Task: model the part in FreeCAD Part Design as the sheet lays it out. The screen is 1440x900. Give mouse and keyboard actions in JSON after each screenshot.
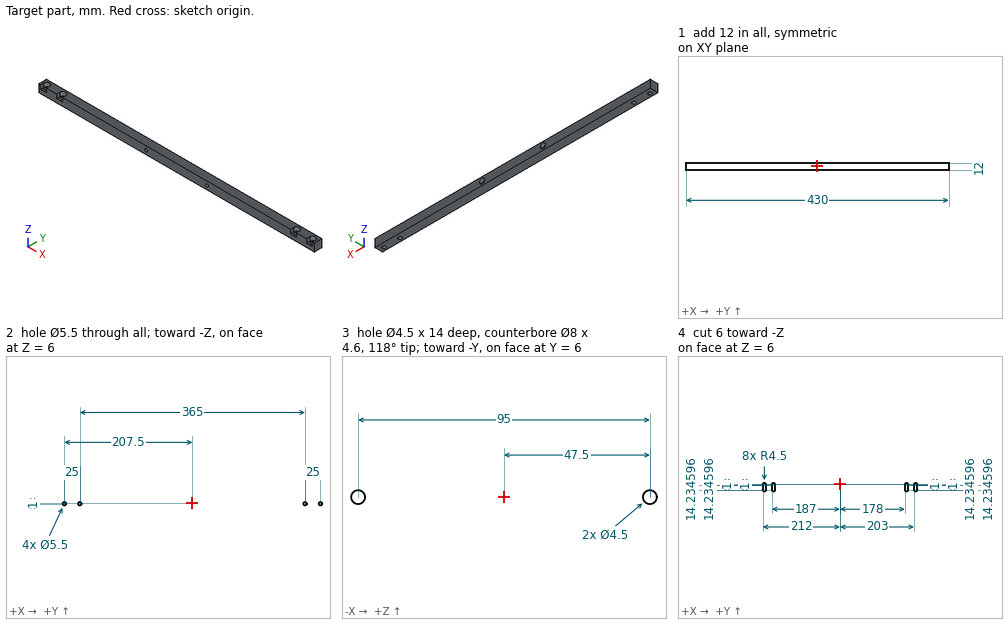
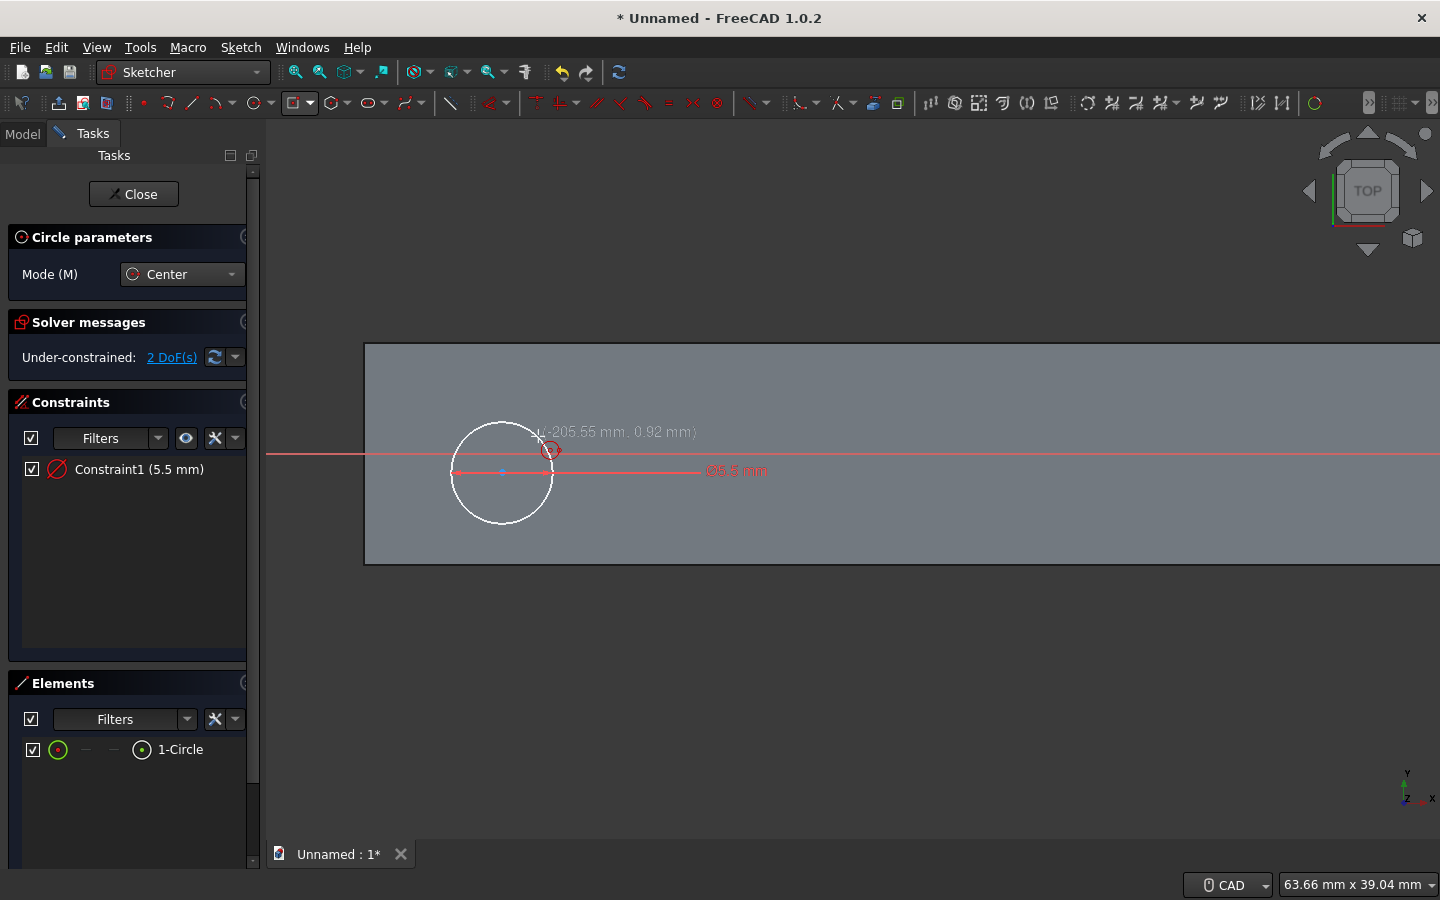
{"action": "left_click", "coordinate": [963, 472]}
{"action": "mouse_move", "coordinate": [999, 436]}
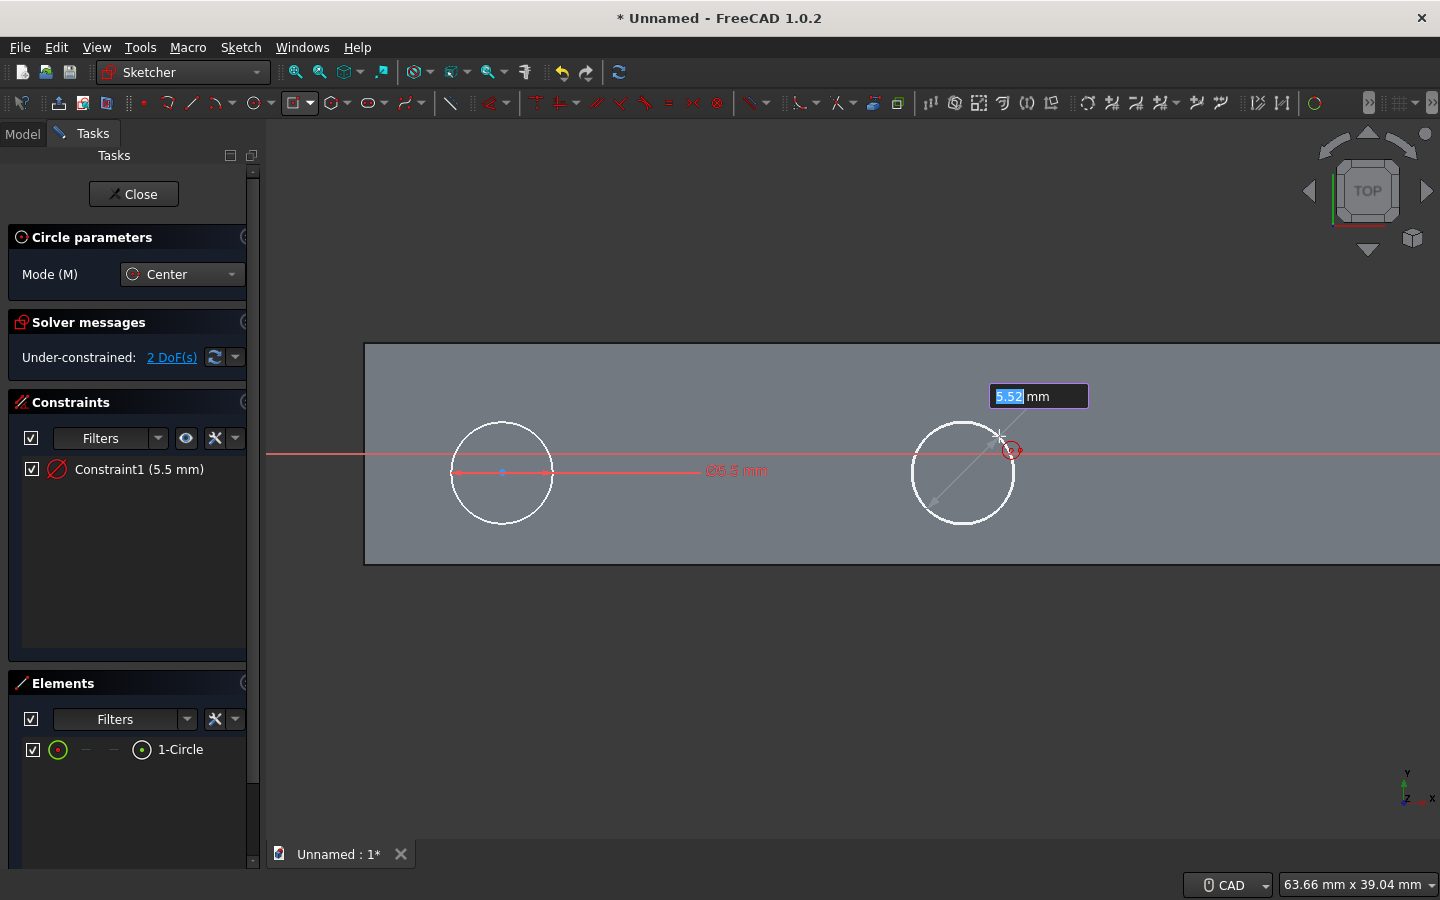
{"action": "type", "text": "5.5"}
{"action": "key", "text": "Return"}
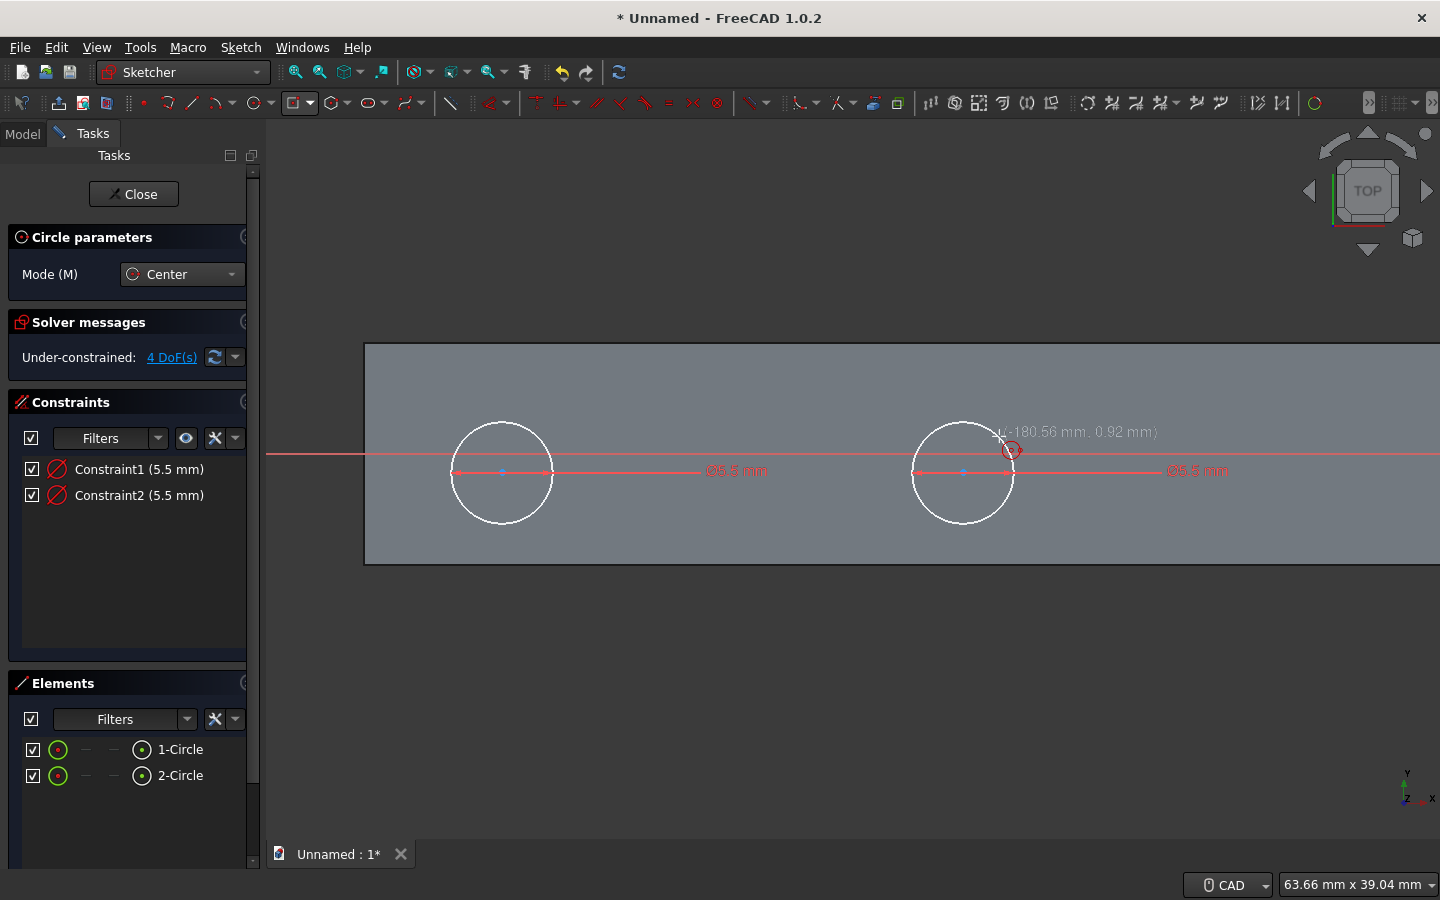
{"action": "scroll", "coordinate": [431, 480], "scroll_direction": "down", "scroll_amount": 12}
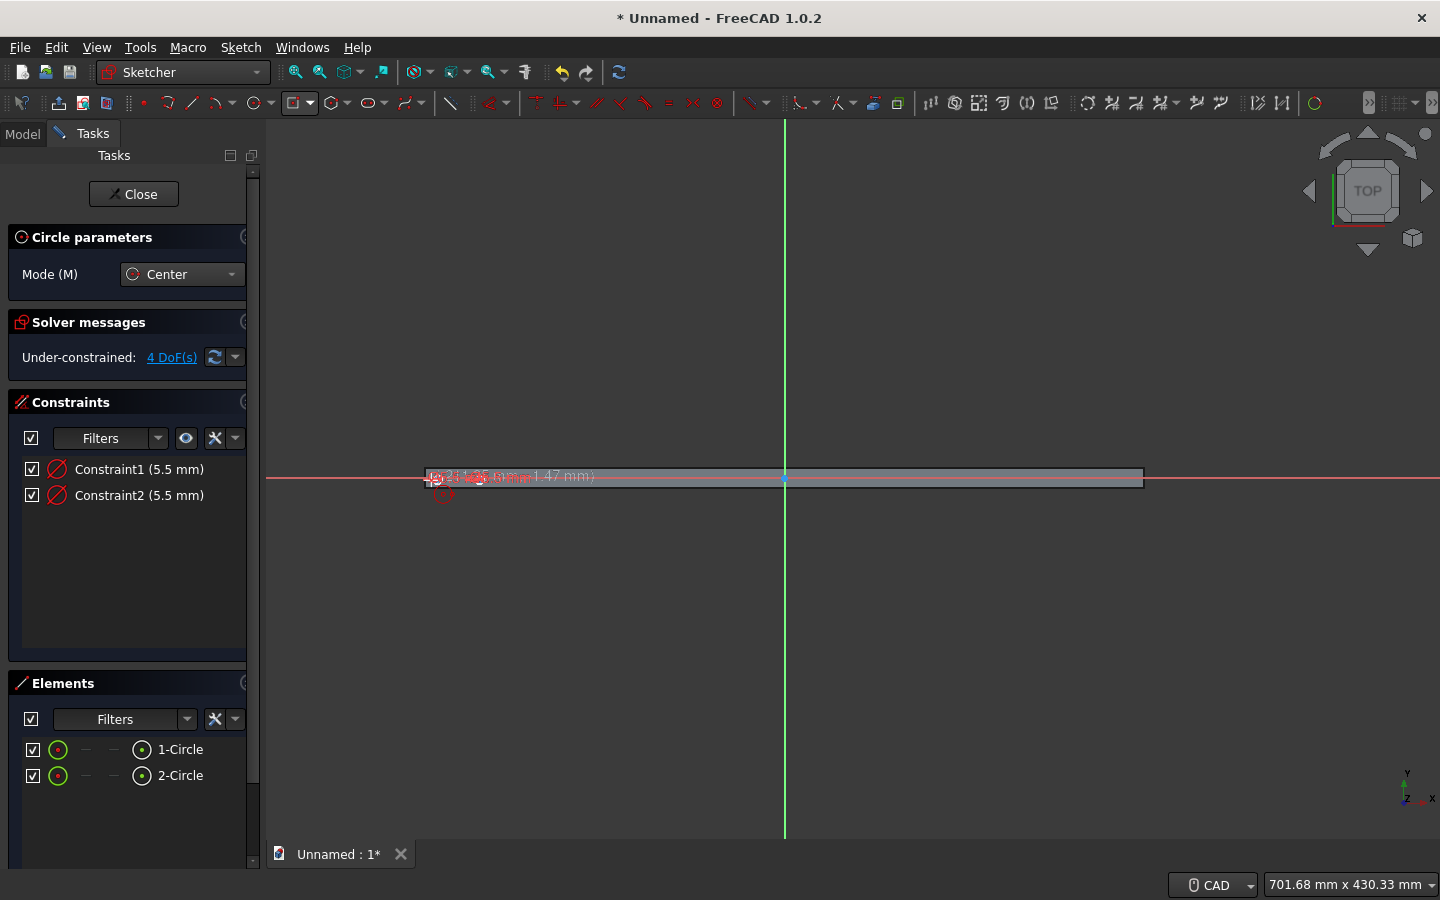
{"action": "scroll", "coordinate": [1090, 480], "scroll_direction": "up", "scroll_amount": 12}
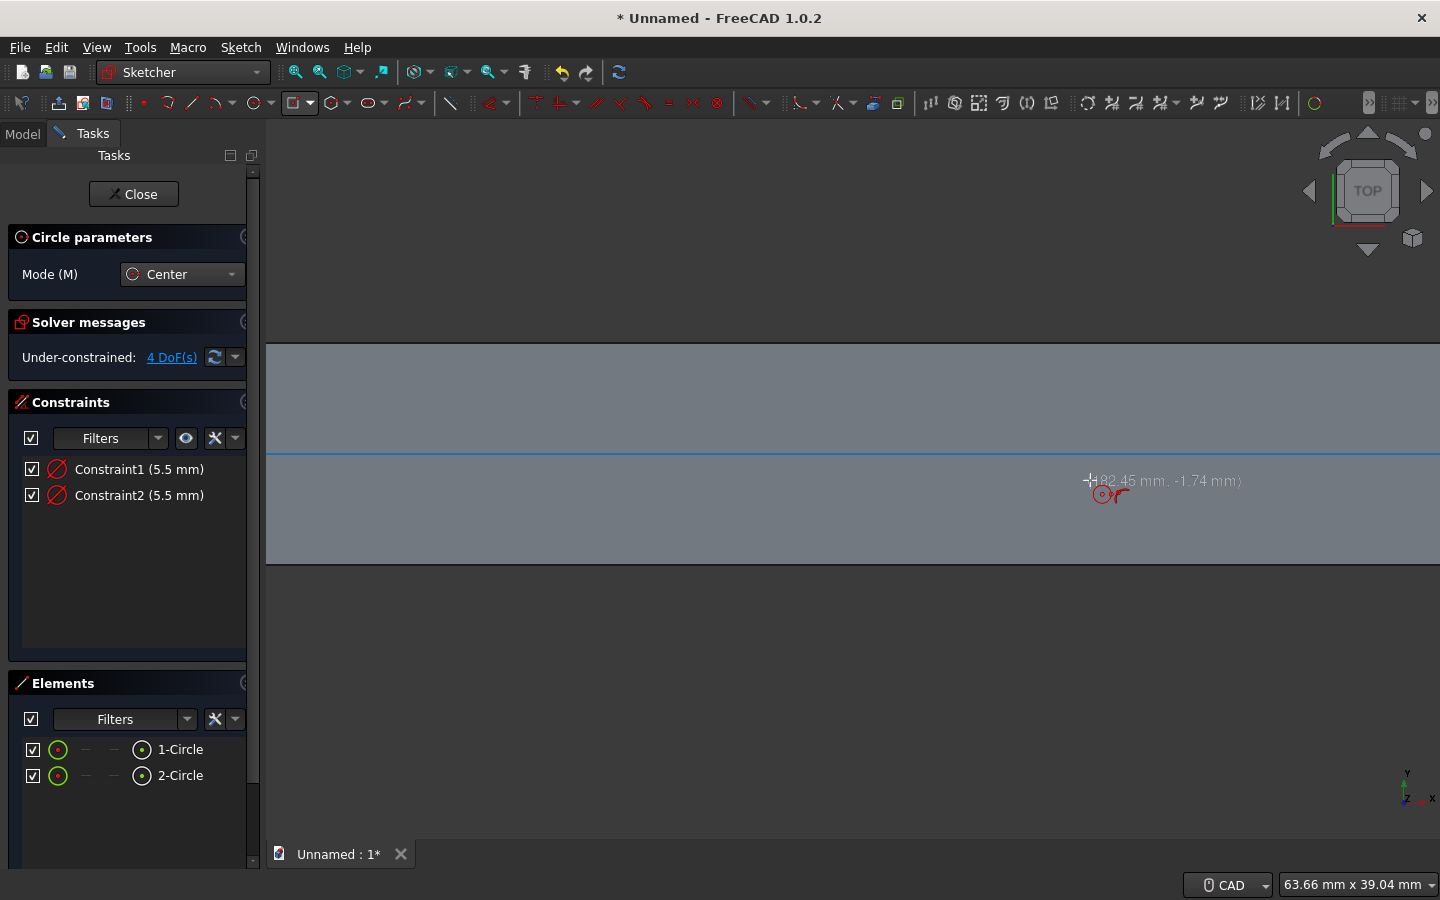
{"action": "left_click", "coordinate": [1084, 472]}
{"action": "mouse_move", "coordinate": [1120, 436]}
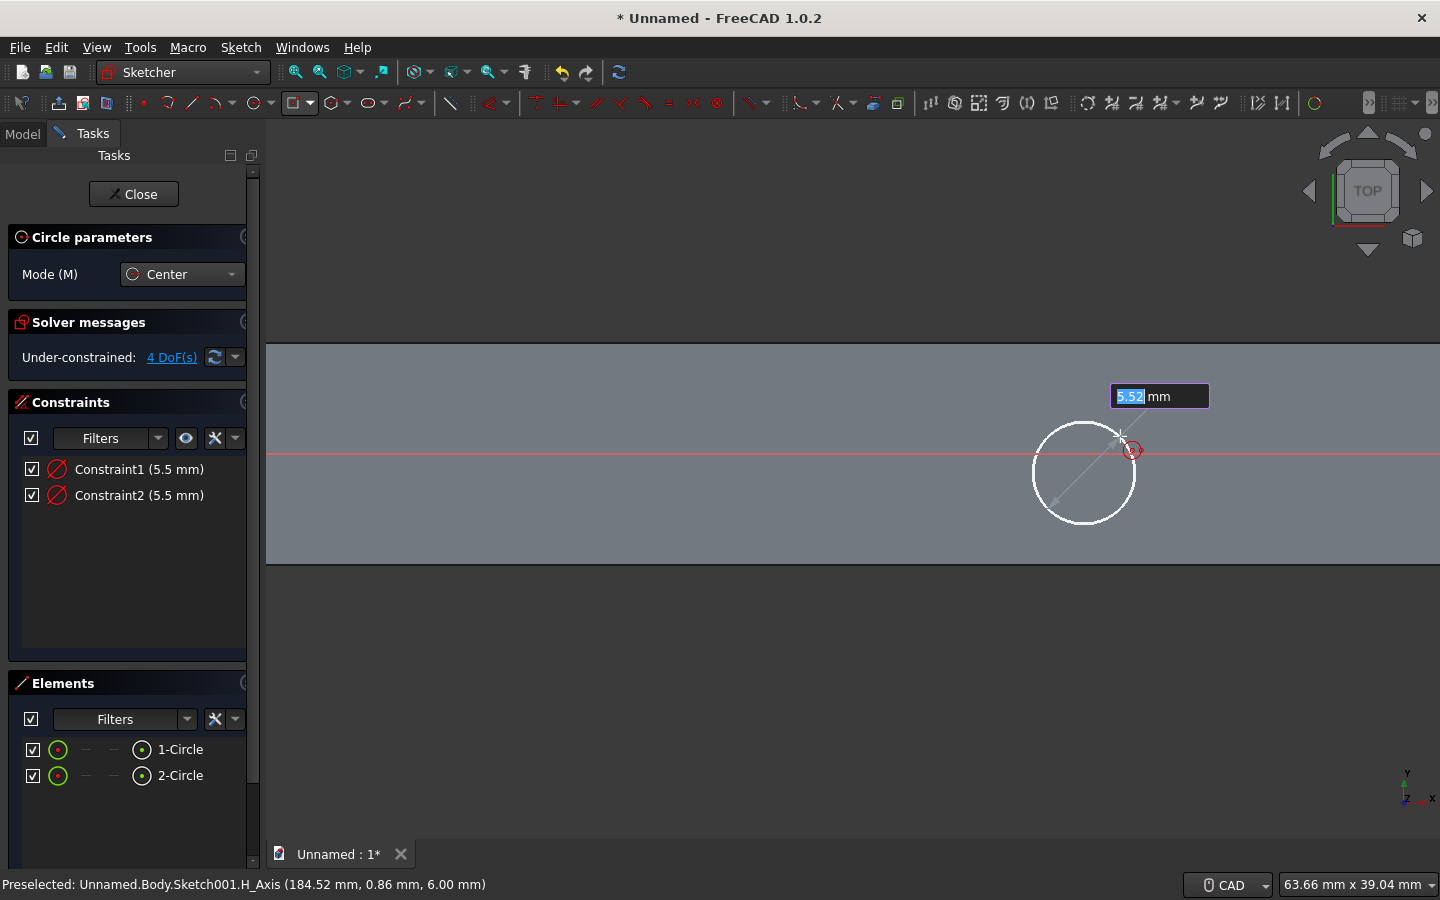
{"action": "type", "text": "5.5"}
{"action": "key", "text": "Return"}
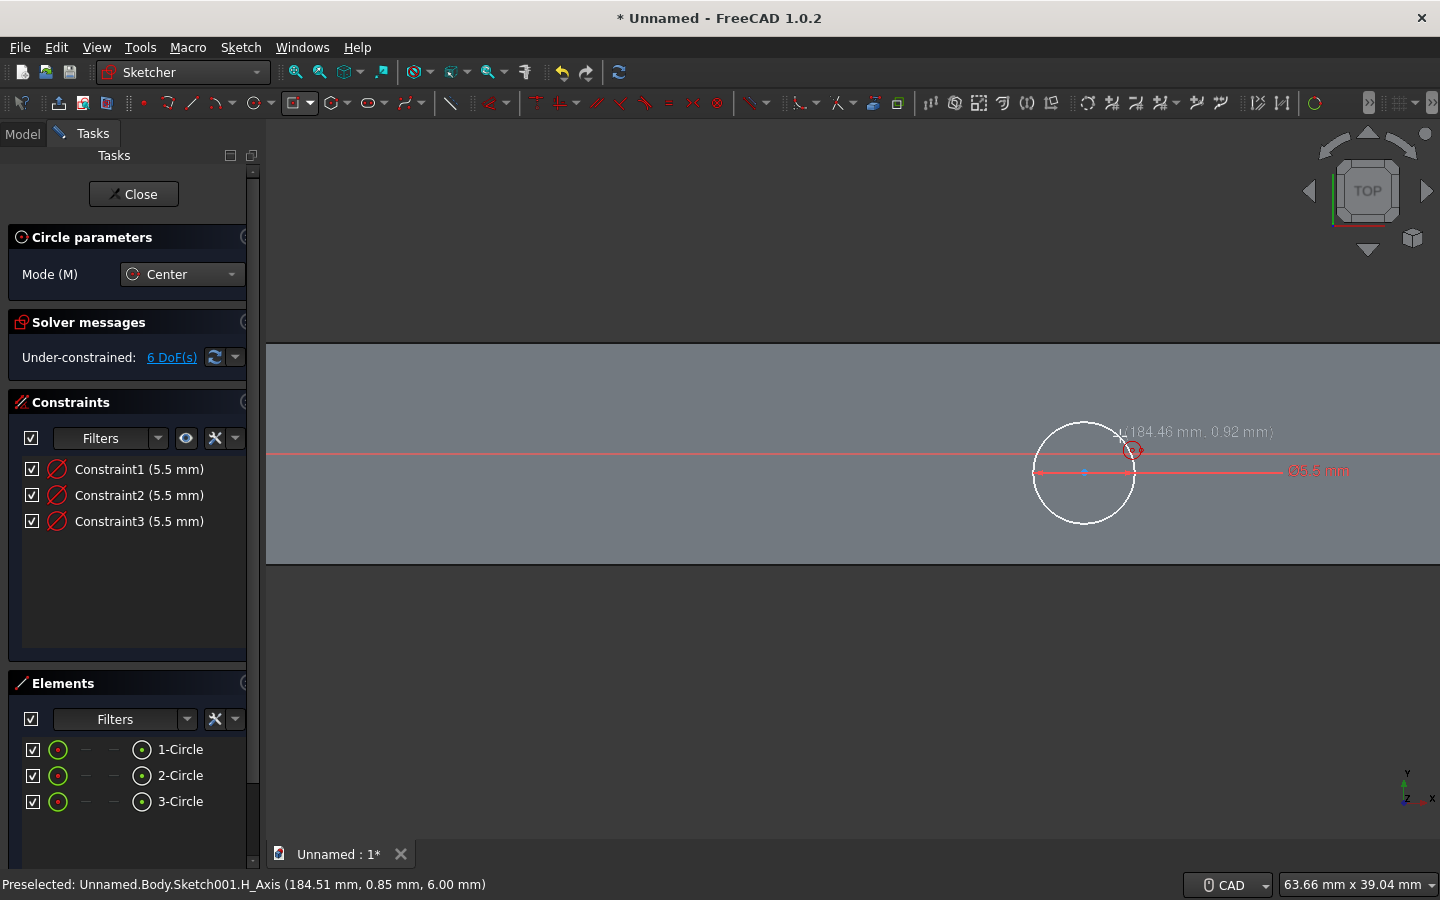
{"action": "scroll", "coordinate": [1090, 480], "scroll_direction": "down", "scroll_amount": 12}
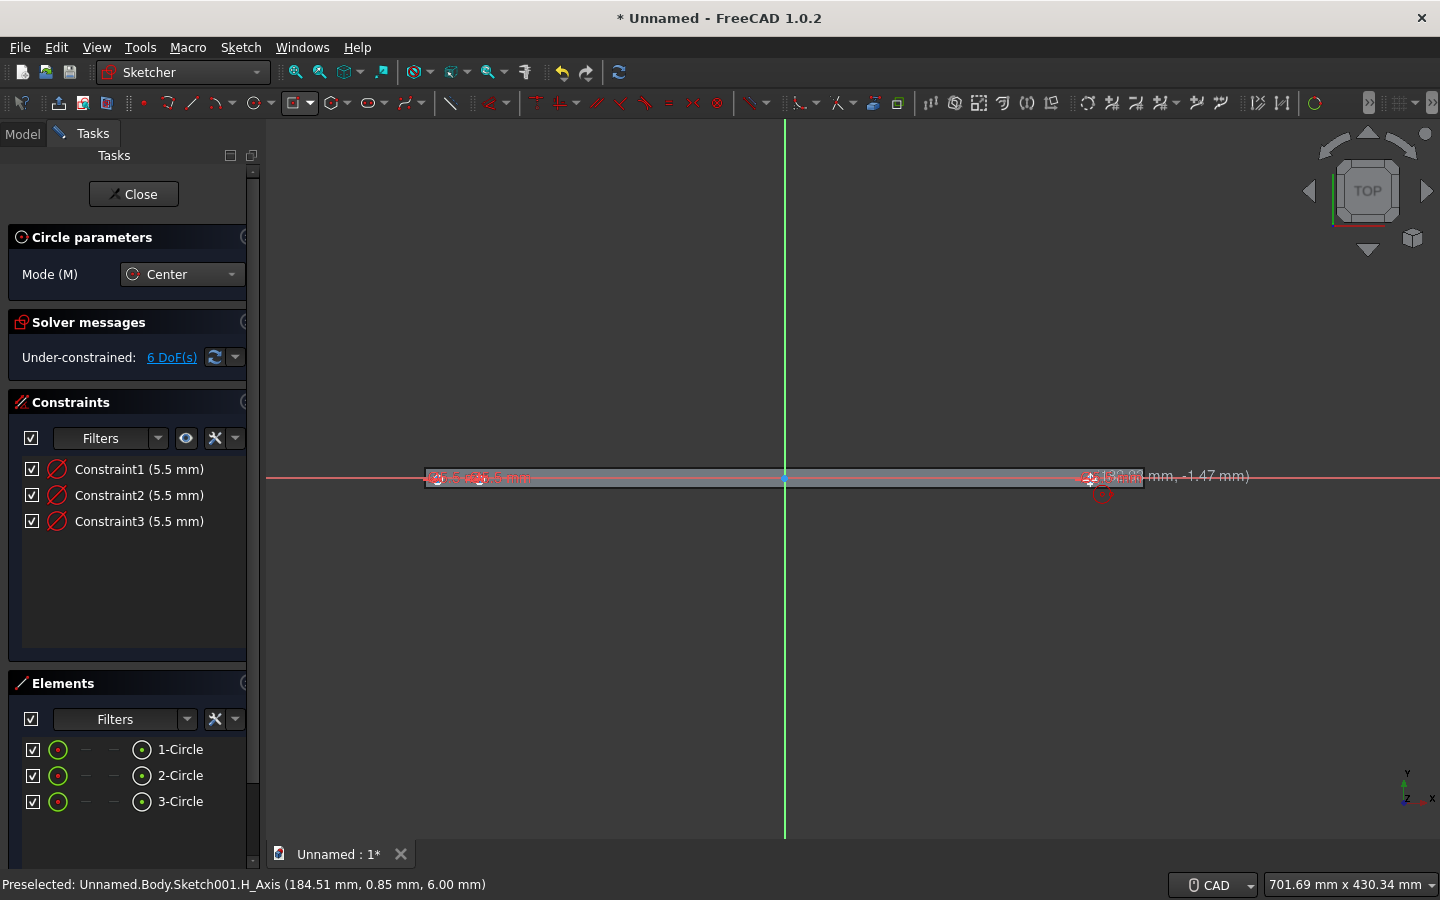
{"action": "scroll", "coordinate": [1132, 480], "scroll_direction": "up", "scroll_amount": 12}